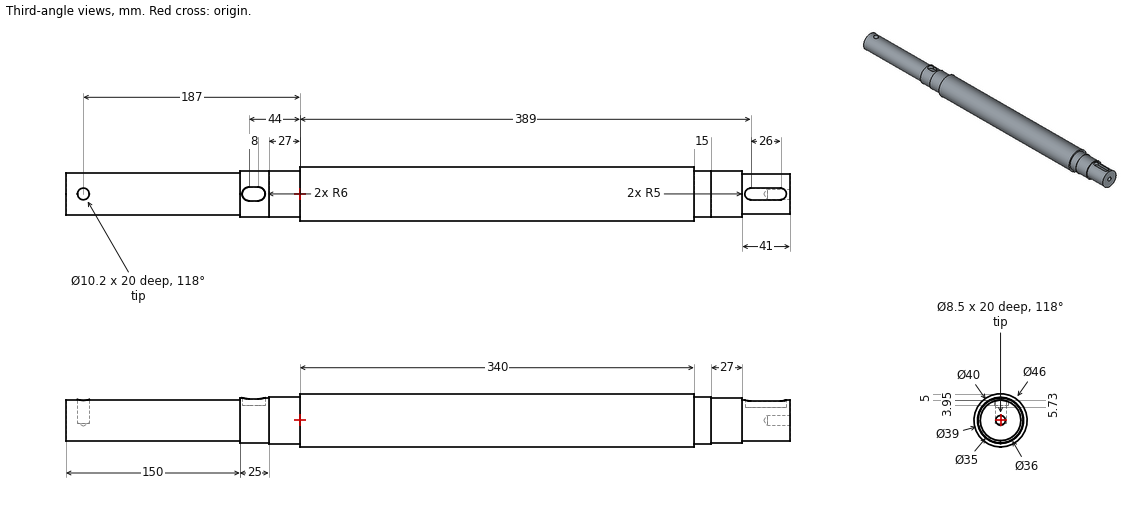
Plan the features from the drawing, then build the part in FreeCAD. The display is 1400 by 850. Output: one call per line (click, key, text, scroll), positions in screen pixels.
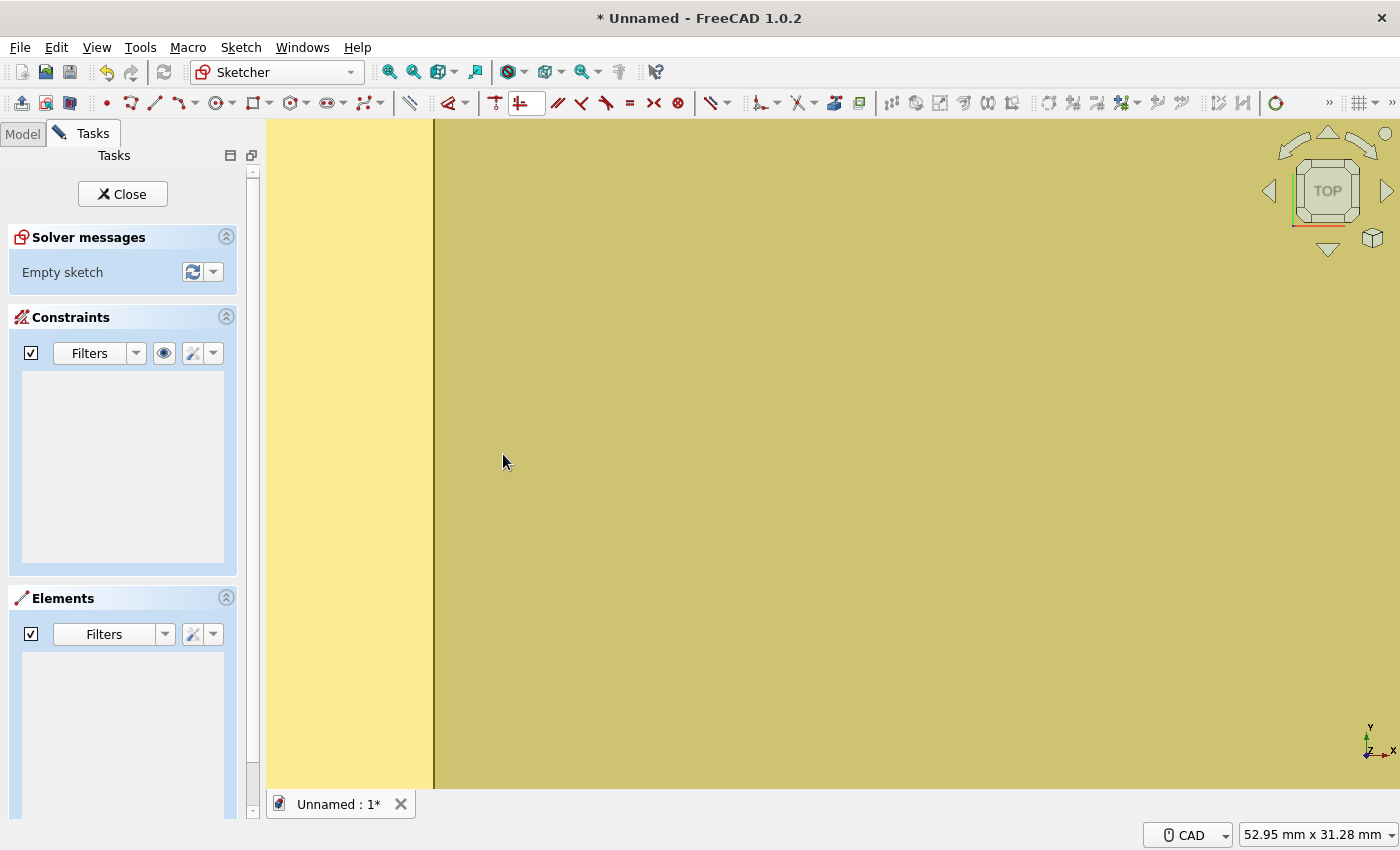
scroll(745, 433, up, 3)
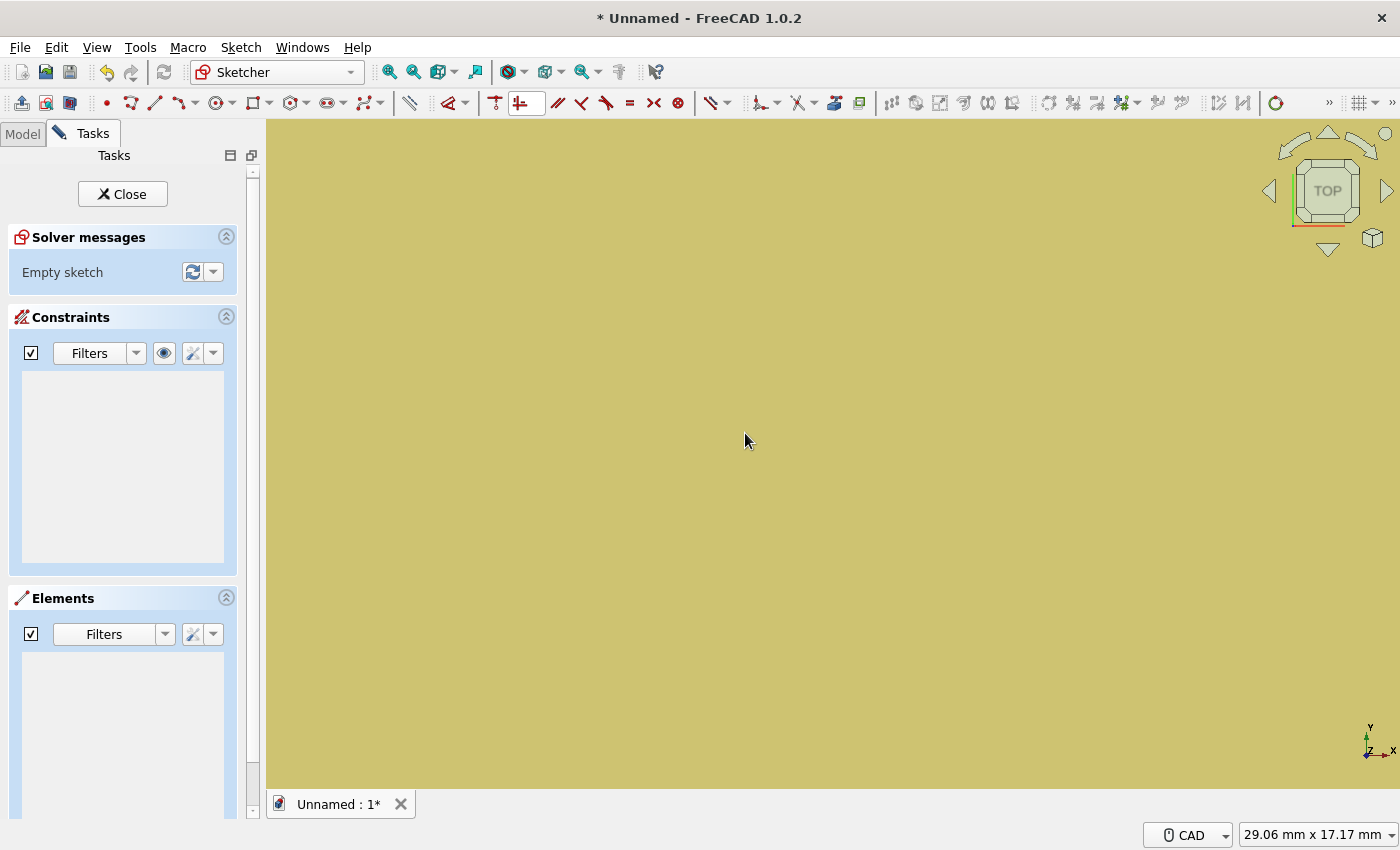
click(216, 104)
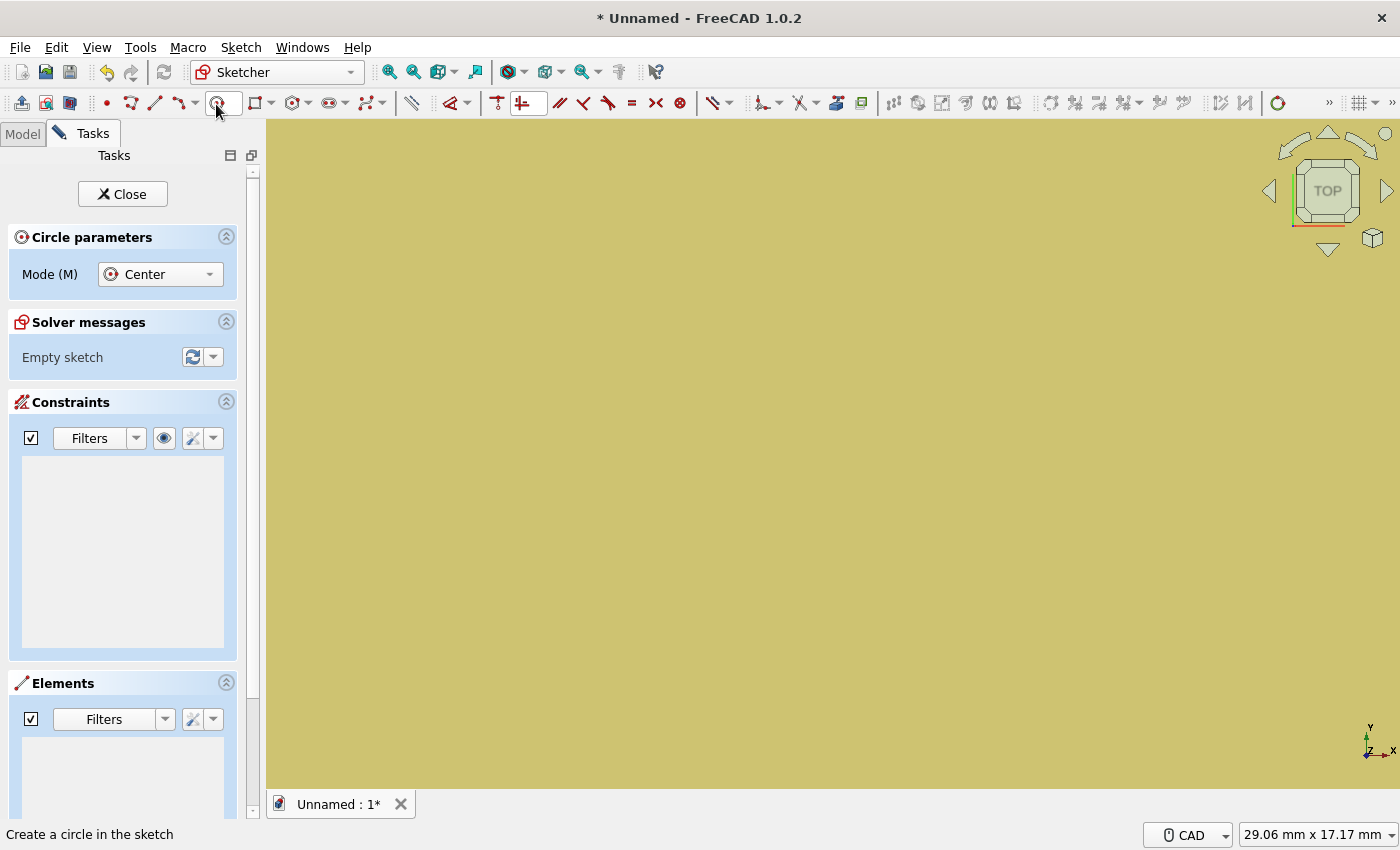
click(764, 453)
click(905, 313)
key(Escape)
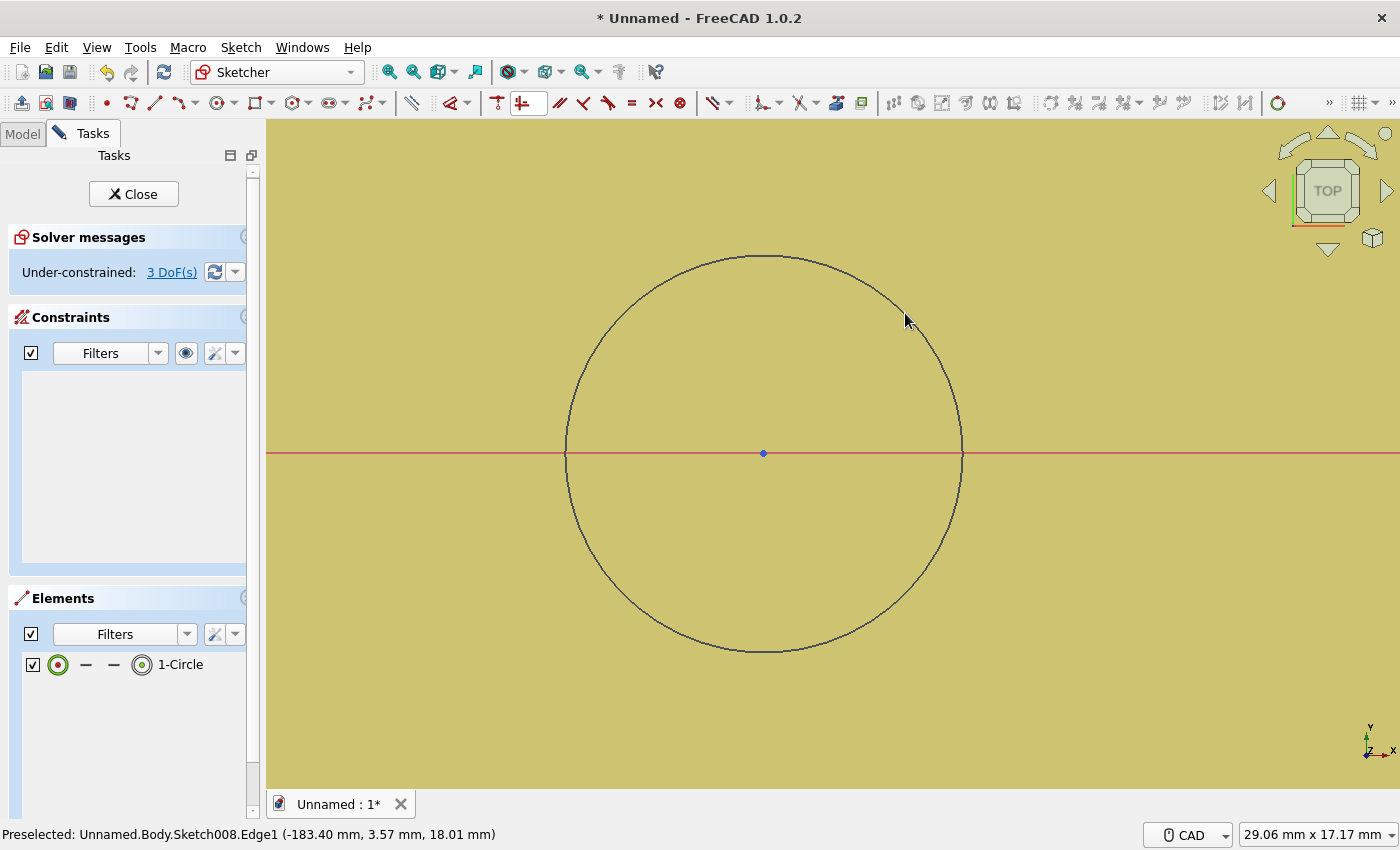
click(764, 454)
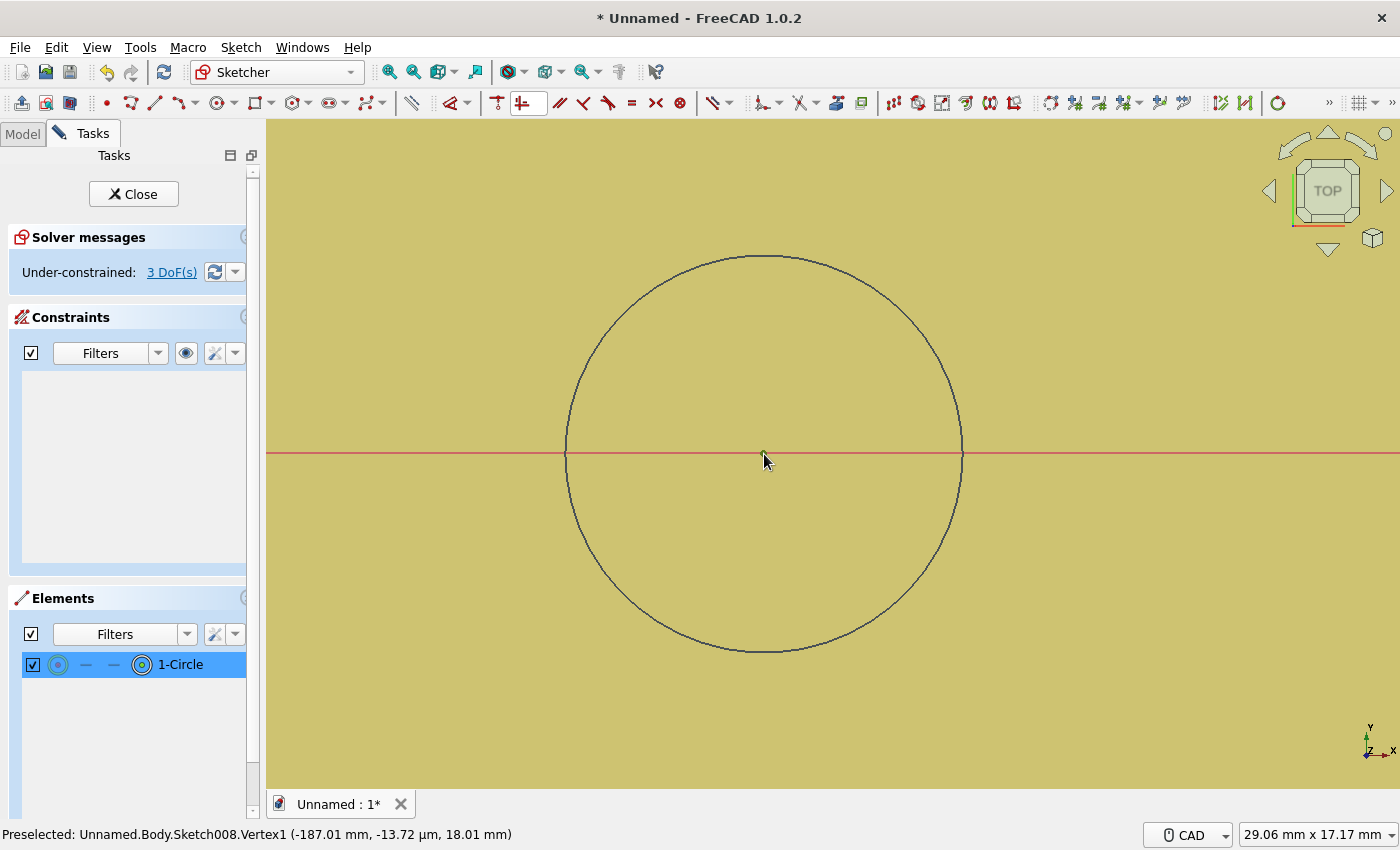
click(361, 453)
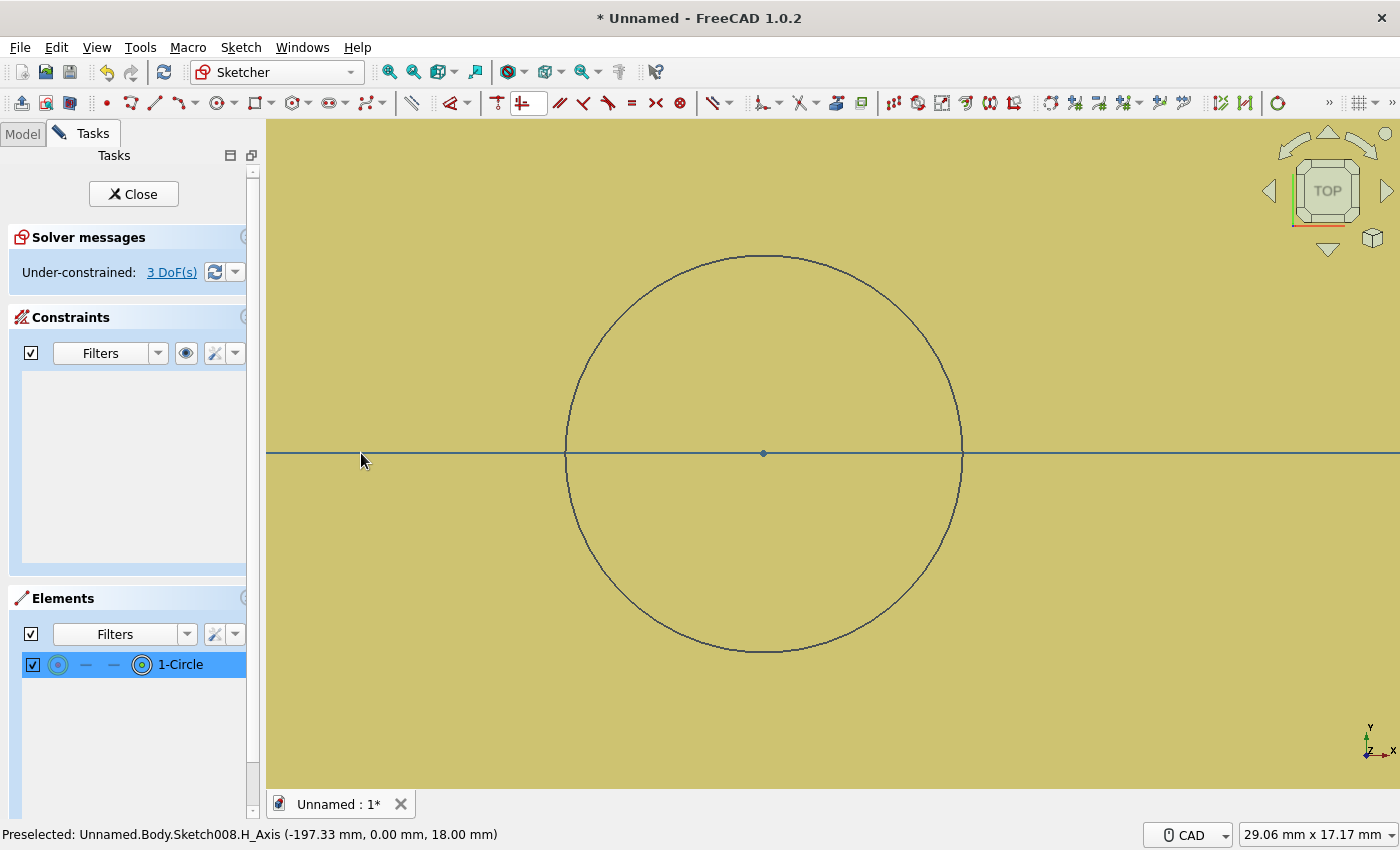
click(498, 104)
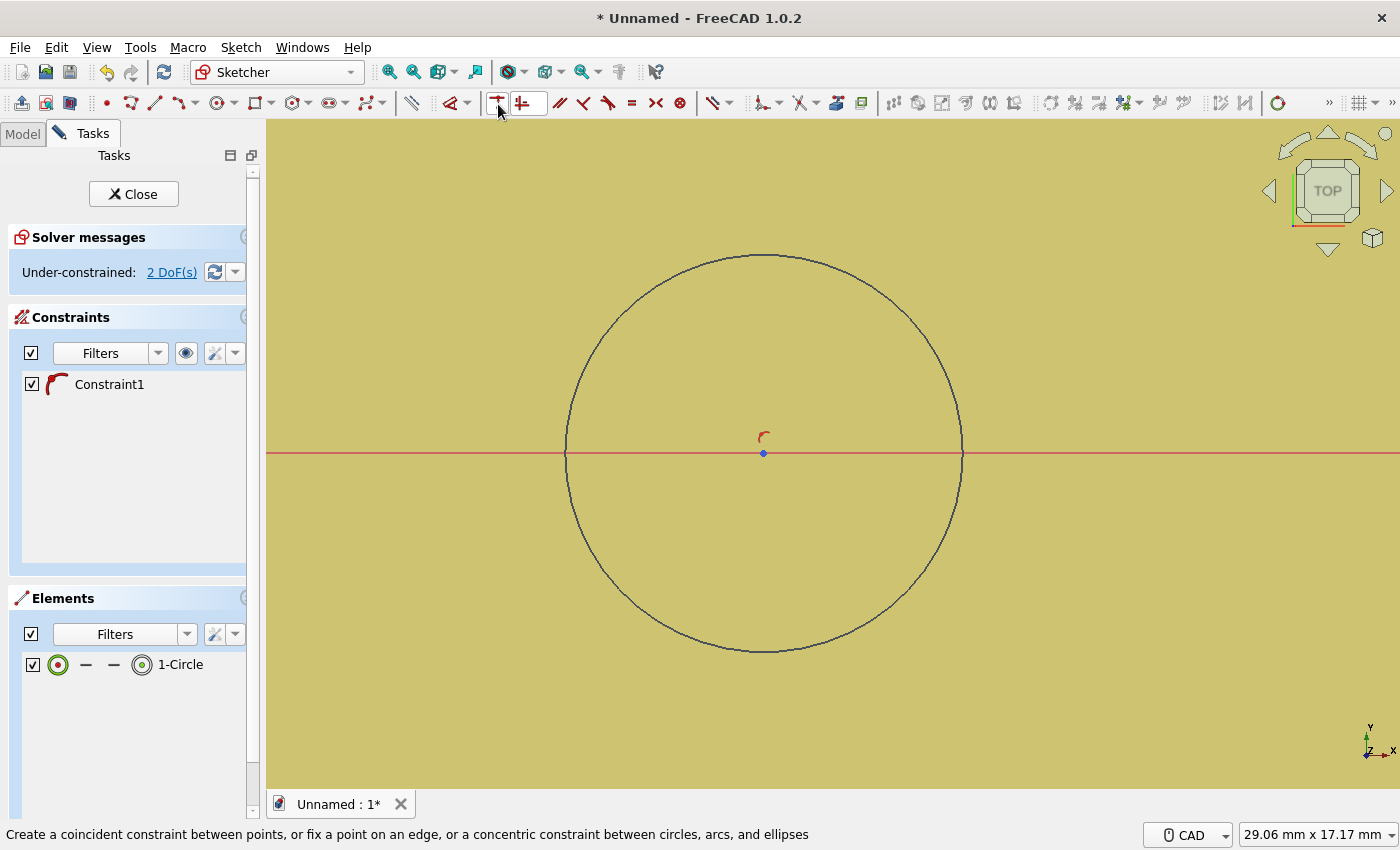
click(450, 104)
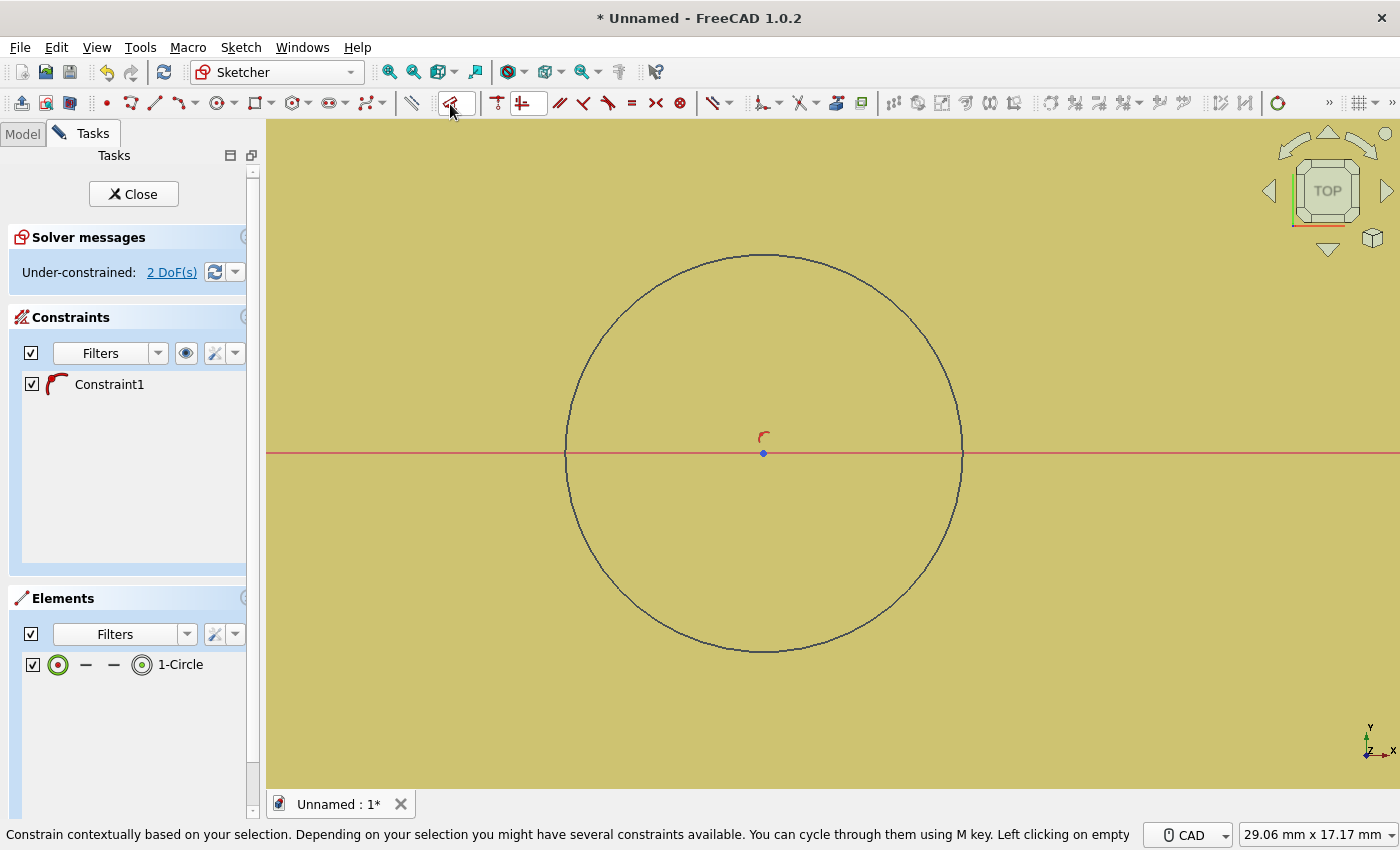
click(904, 313)
click(927, 290)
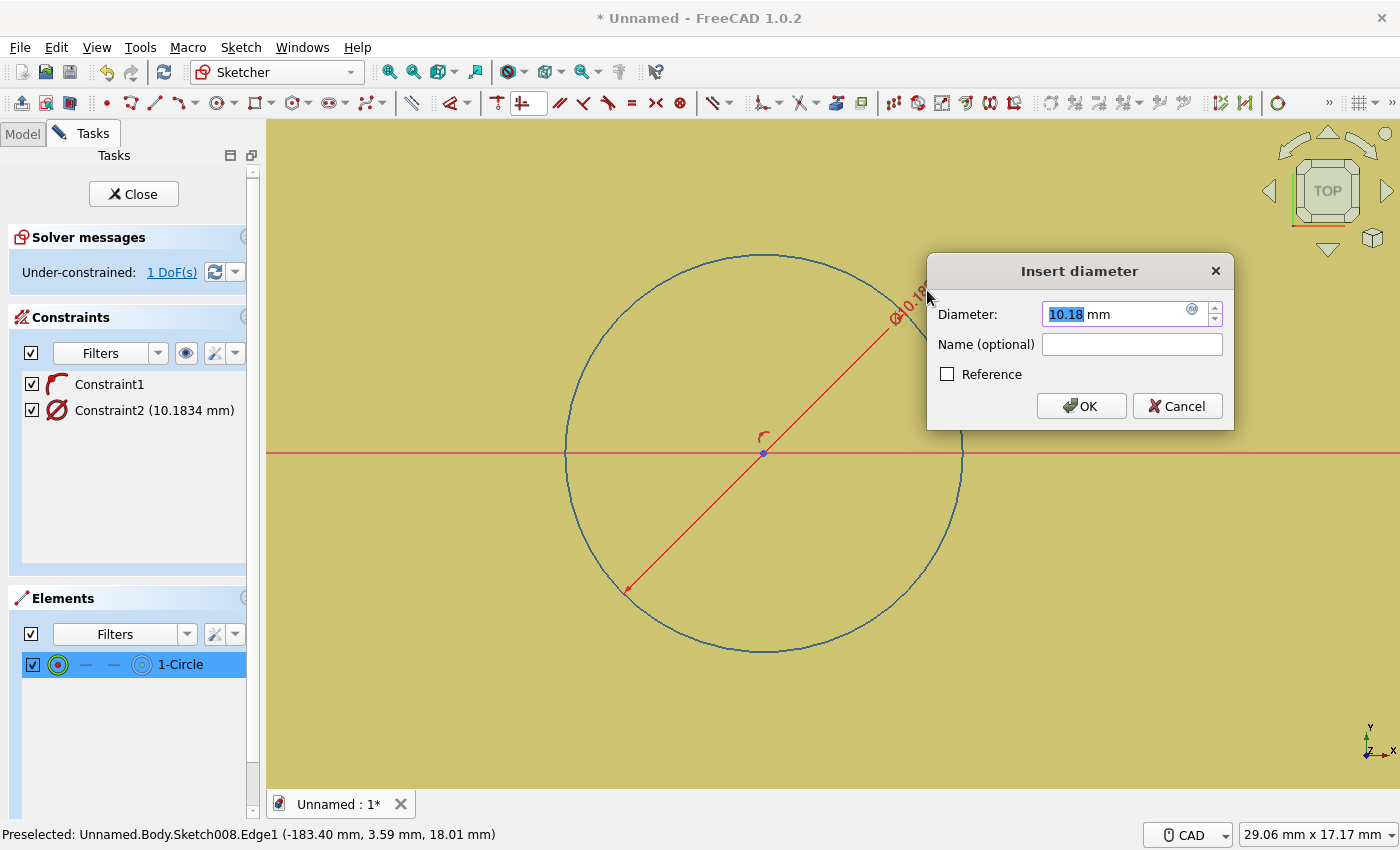
text(10.2)
key(Return)